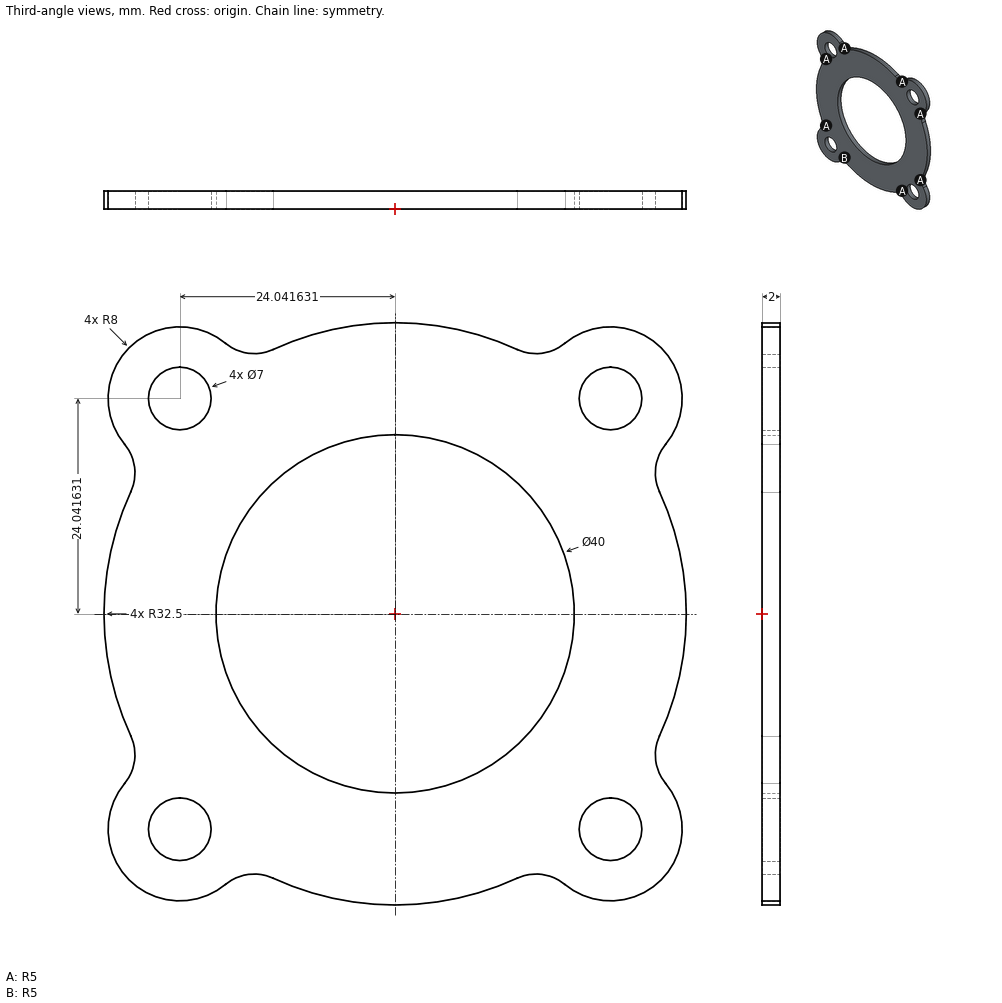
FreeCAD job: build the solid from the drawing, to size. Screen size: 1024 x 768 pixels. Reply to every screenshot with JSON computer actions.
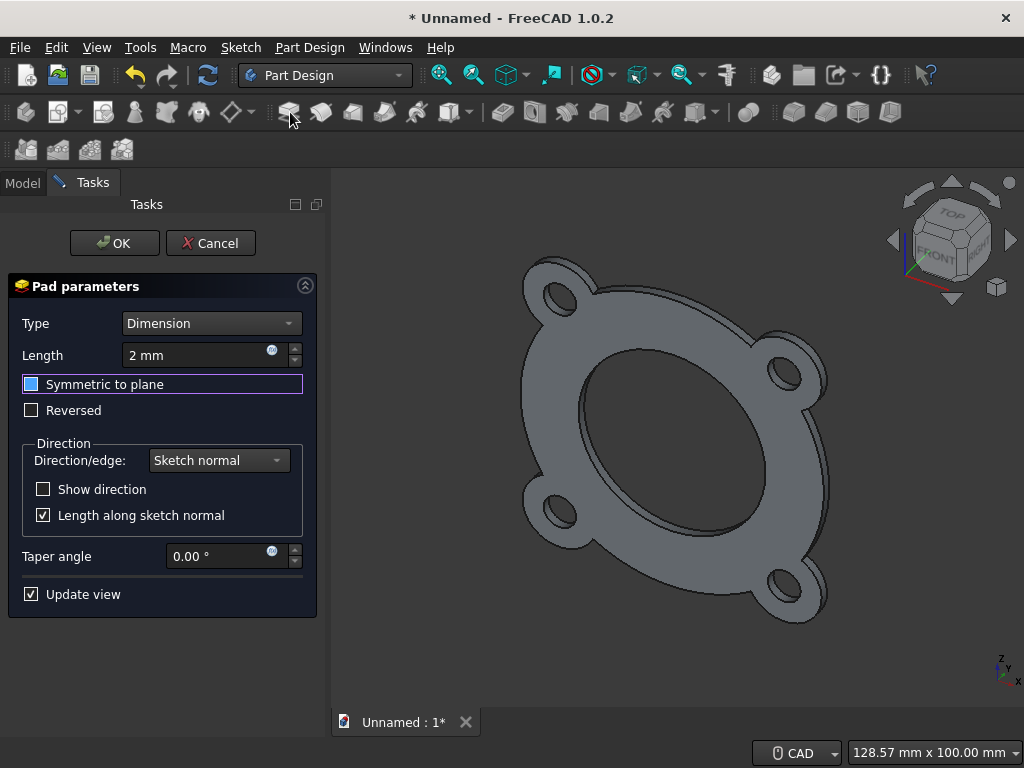
{"action": "left_click", "coordinate": [30, 410]}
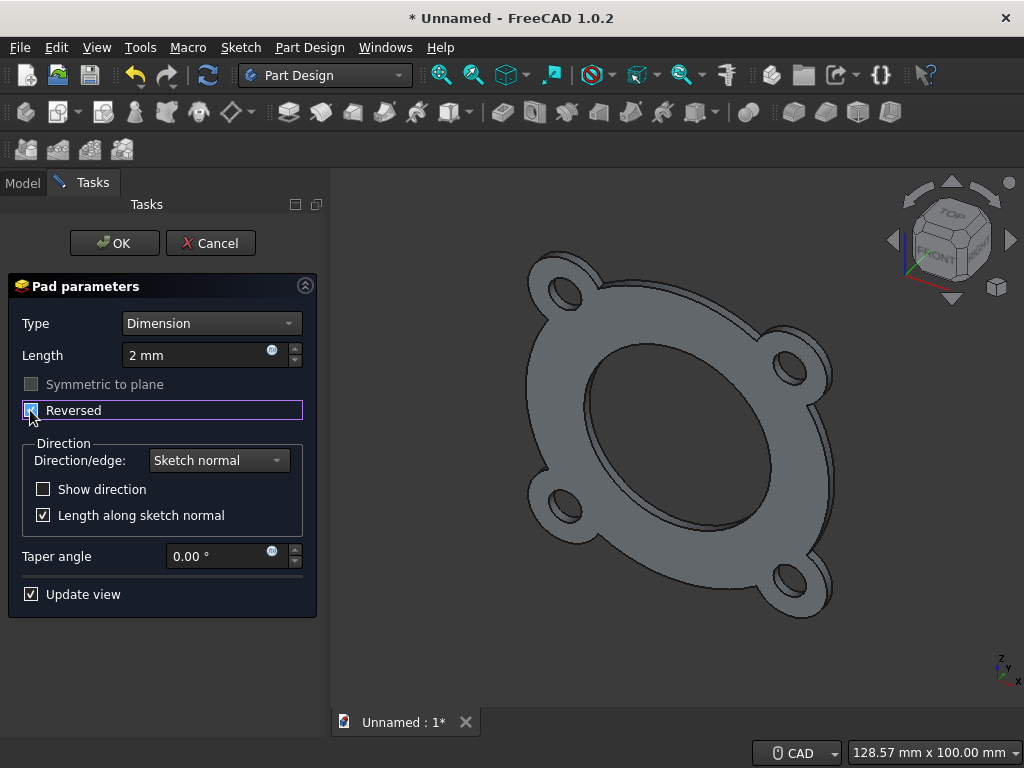
{"action": "left_click", "coordinate": [115, 243]}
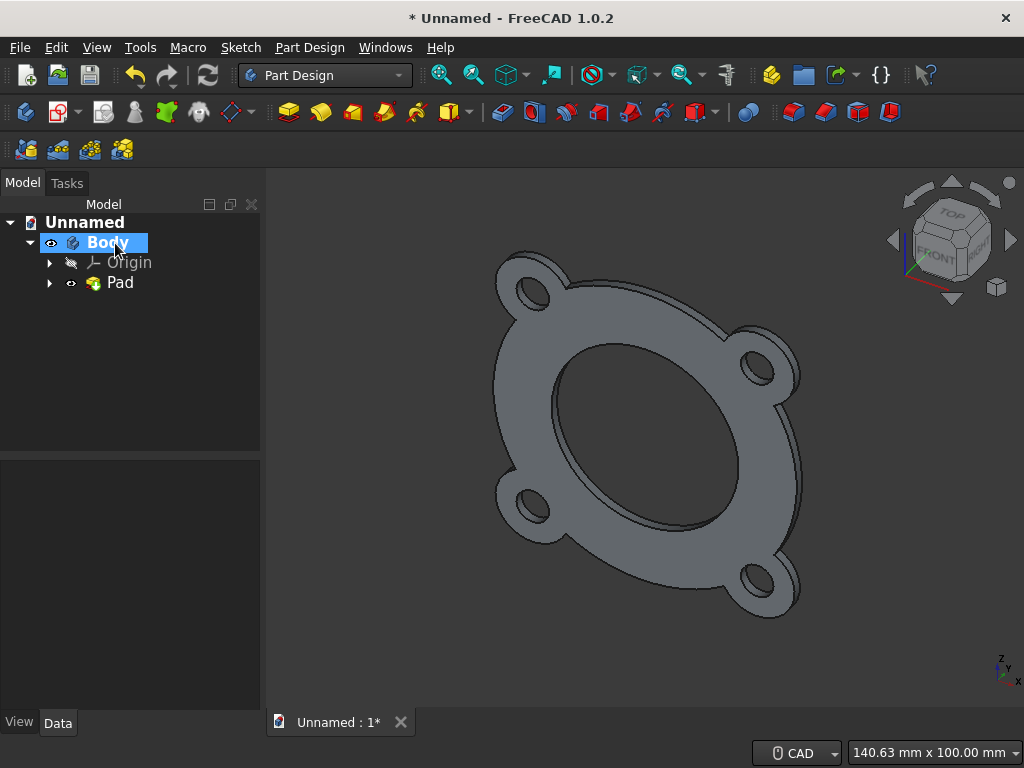
{"action": "scroll", "coordinate": [727, 582], "scroll_direction": "up", "scroll_amount": 7}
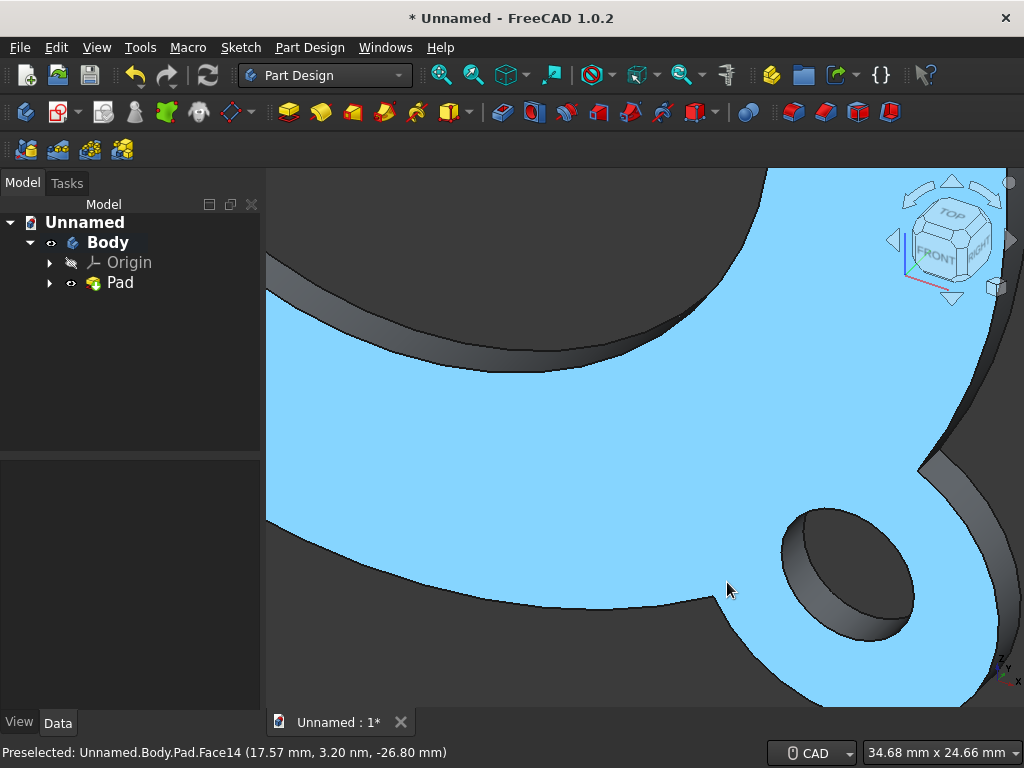
{"action": "left_click", "coordinate": [442, 76]}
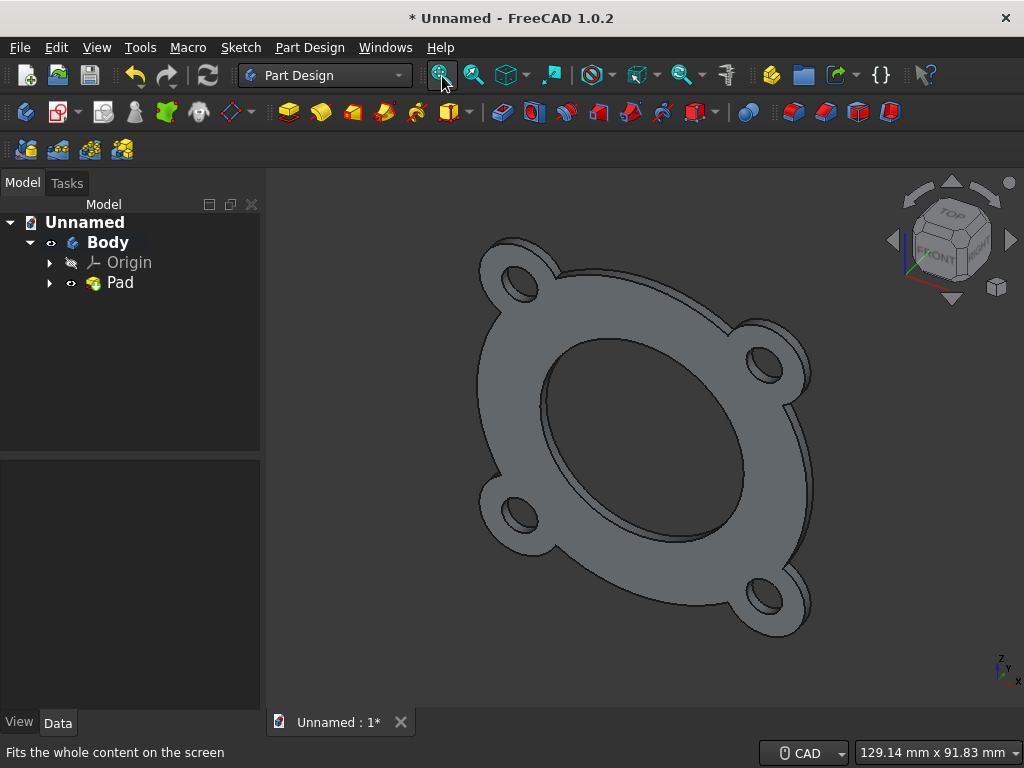
{"action": "key", "text": "0"}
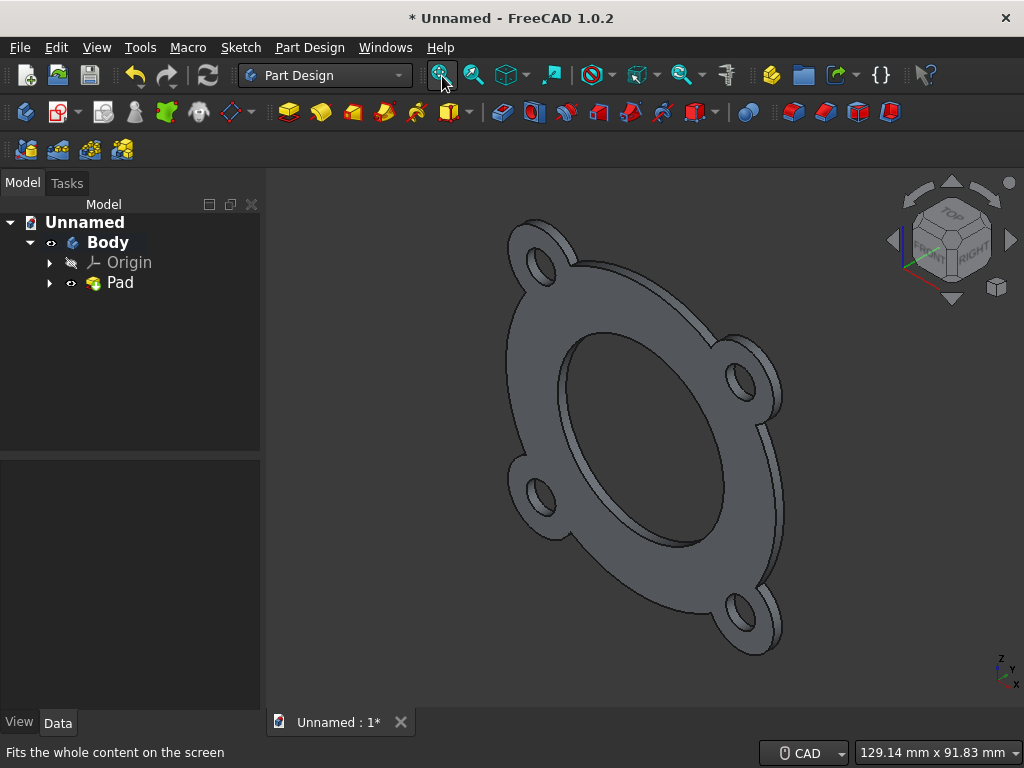
{"action": "scroll", "coordinate": [715, 610], "scroll_direction": "up", "scroll_amount": 7}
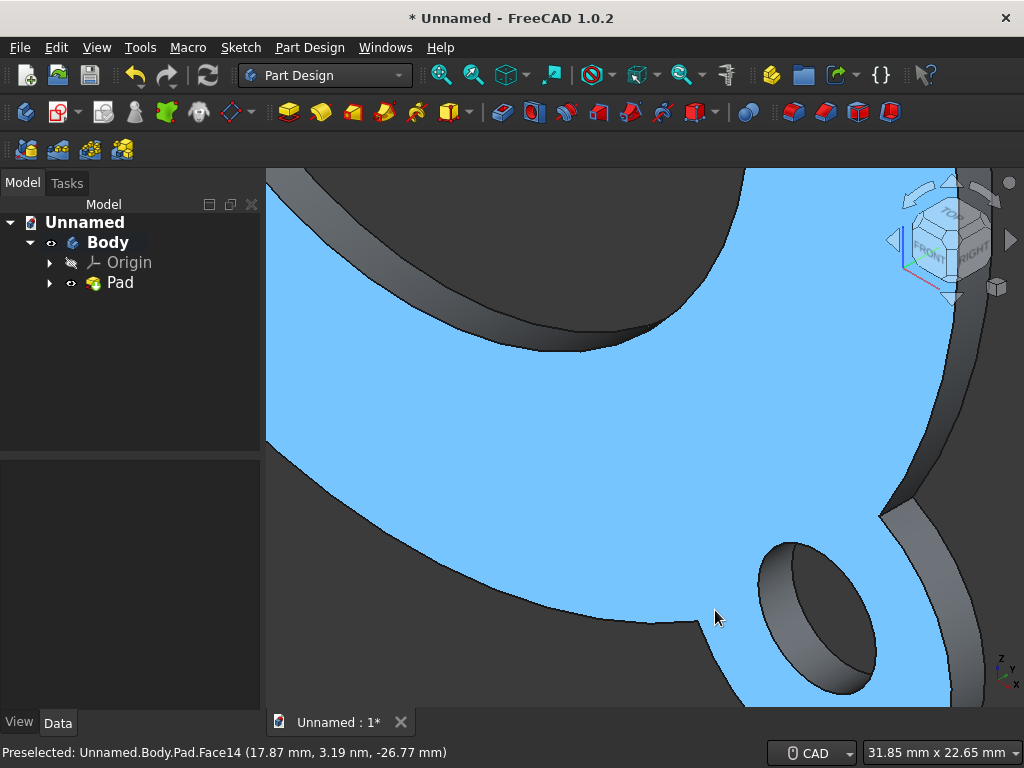
{"action": "left_click", "coordinate": [442, 76]}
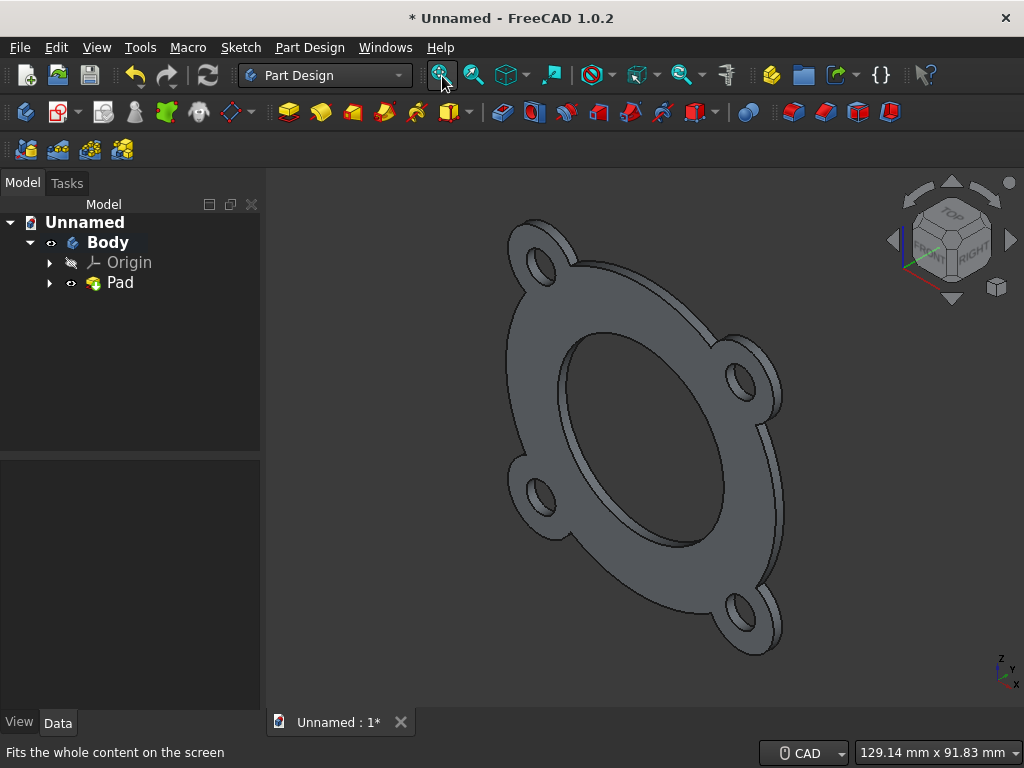
{"action": "key", "text": "2"}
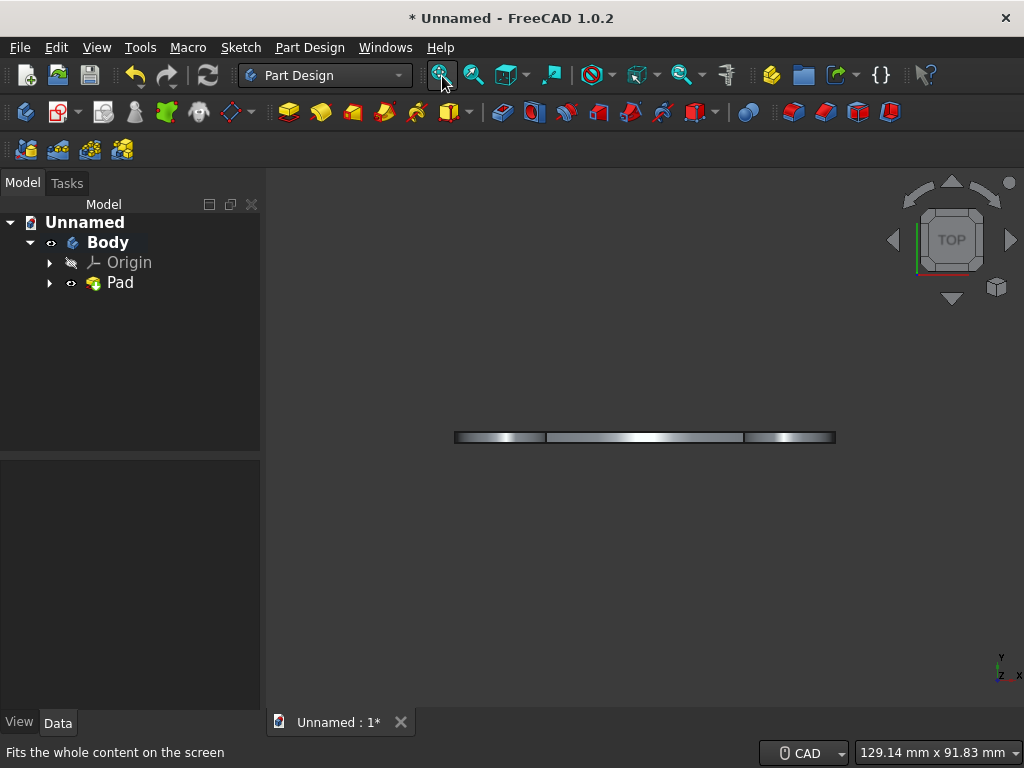
{"action": "scroll", "coordinate": [744, 436], "scroll_direction": "up", "scroll_amount": 7}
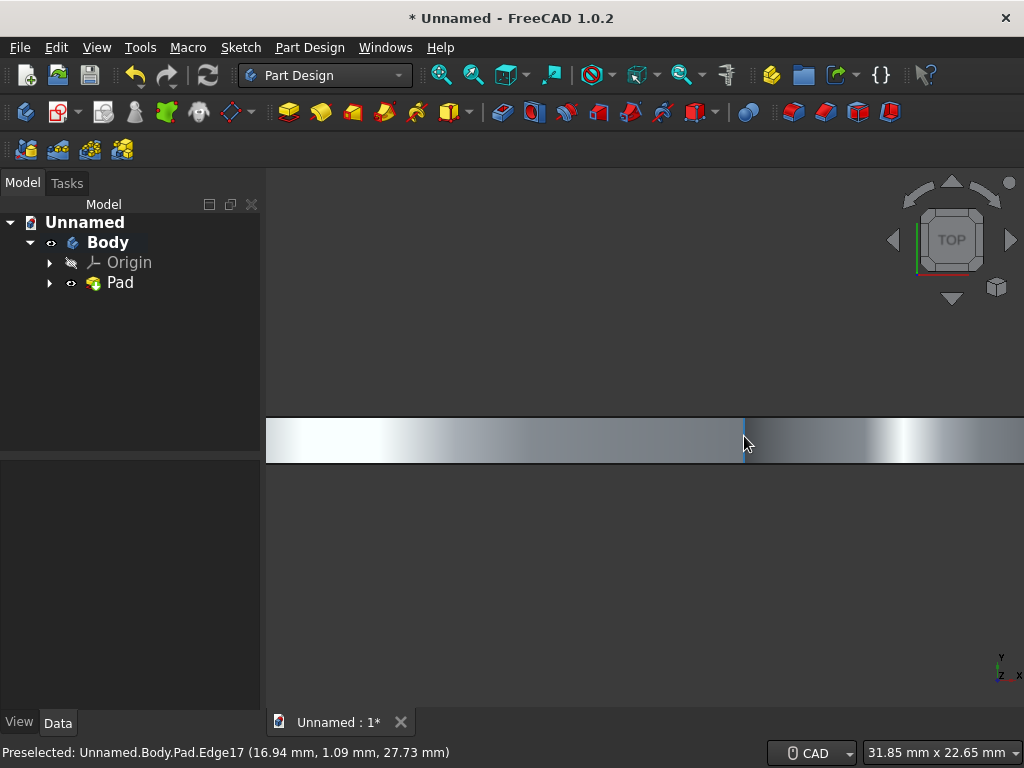
{"action": "left_click", "coordinate": [442, 76]}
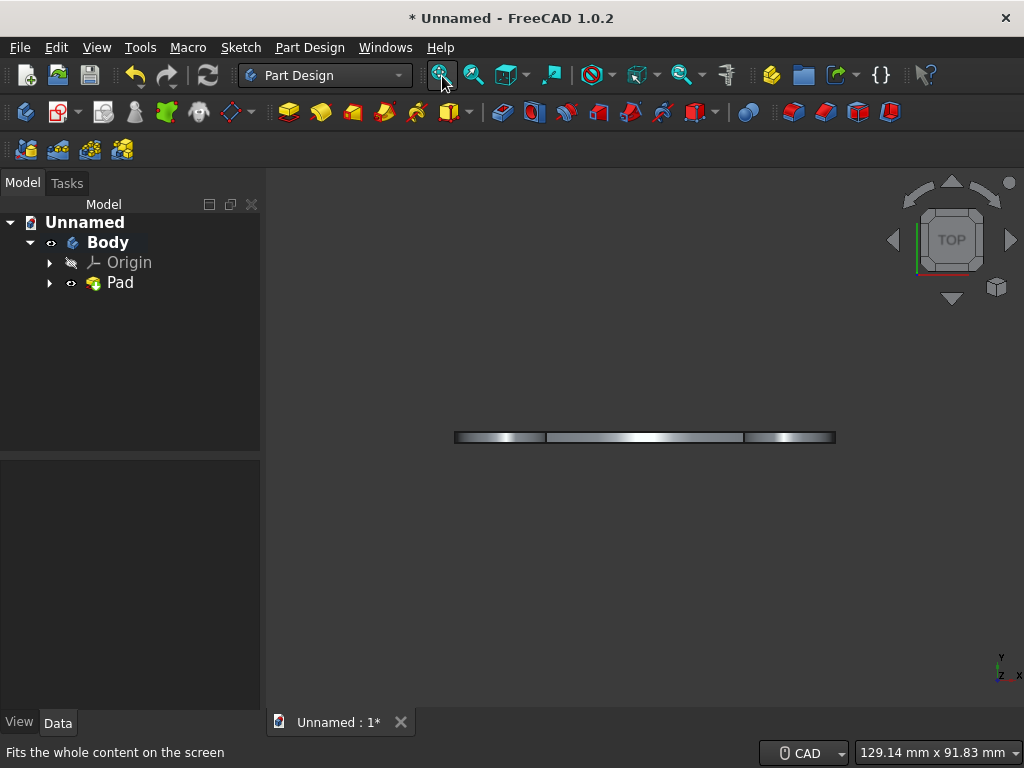
{"action": "key", "text": "1"}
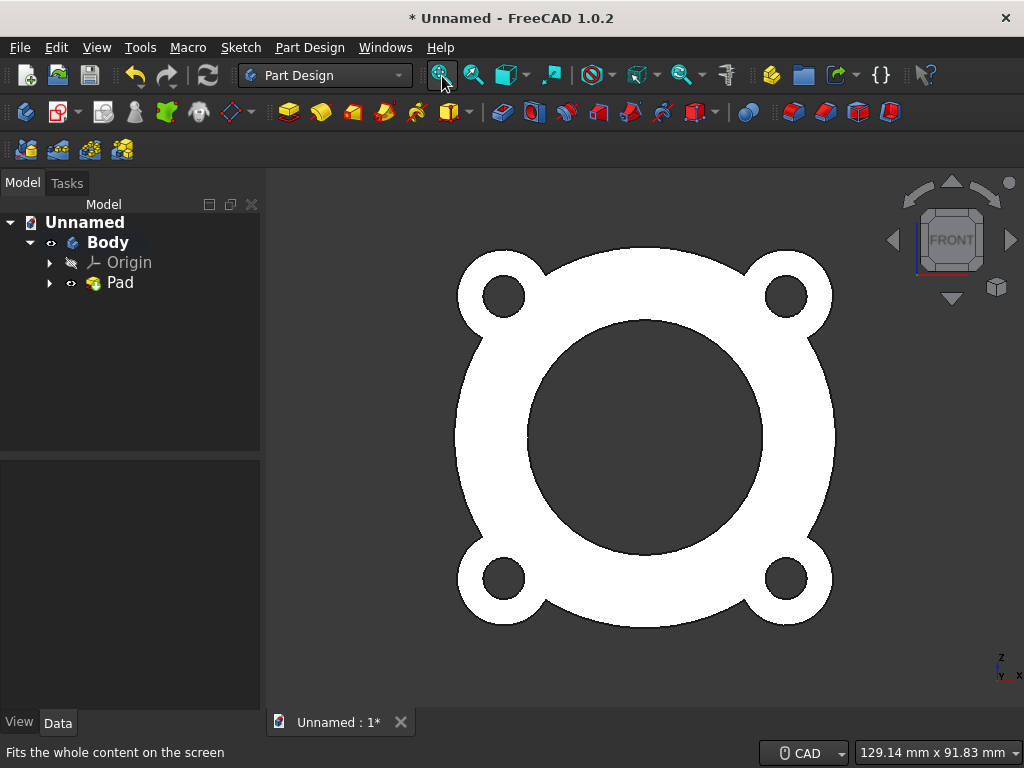
{"action": "scroll", "coordinate": [744, 599], "scroll_direction": "up", "scroll_amount": 7}